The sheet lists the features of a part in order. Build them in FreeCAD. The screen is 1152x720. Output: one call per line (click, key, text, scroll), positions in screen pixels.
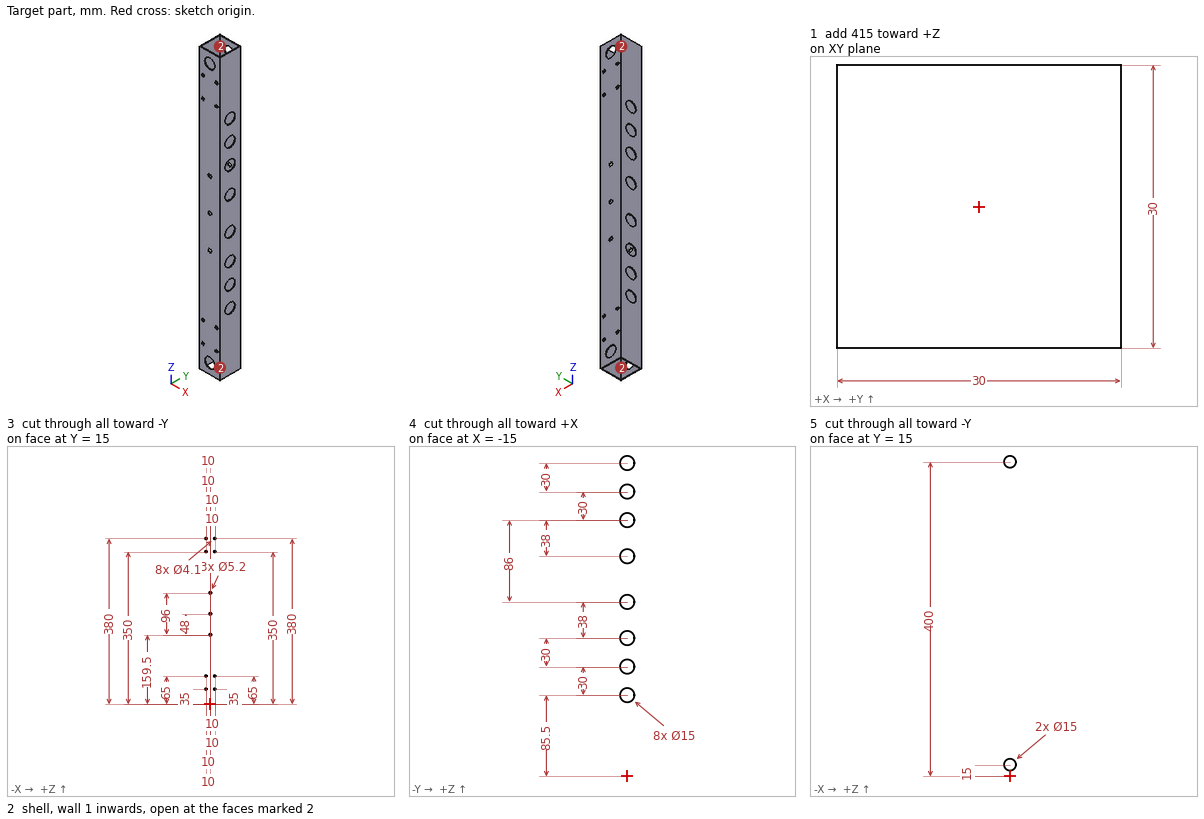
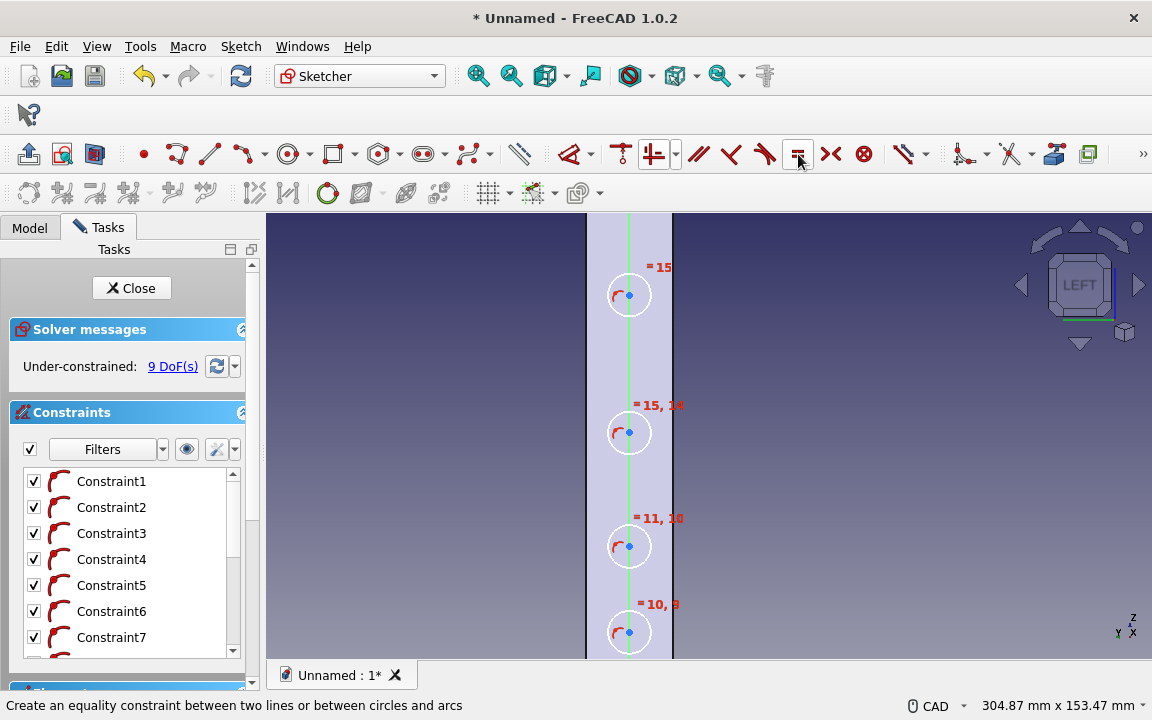
scroll(645, 419, down, 6)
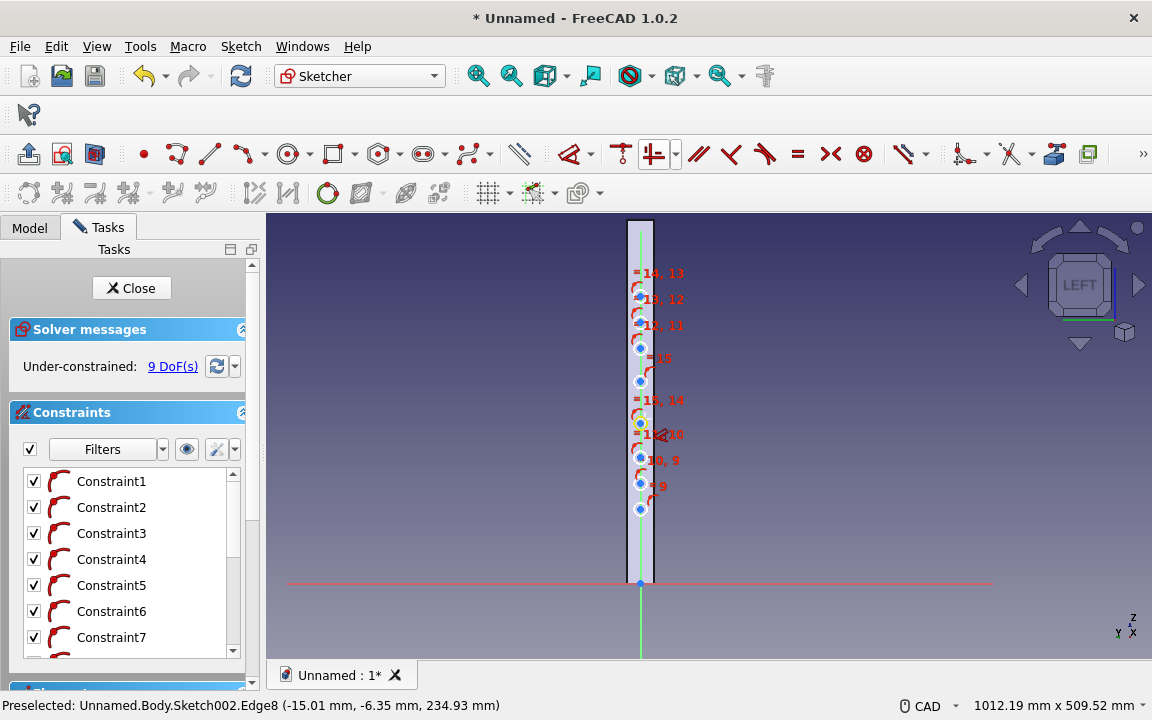
scroll(645, 505, up, 6)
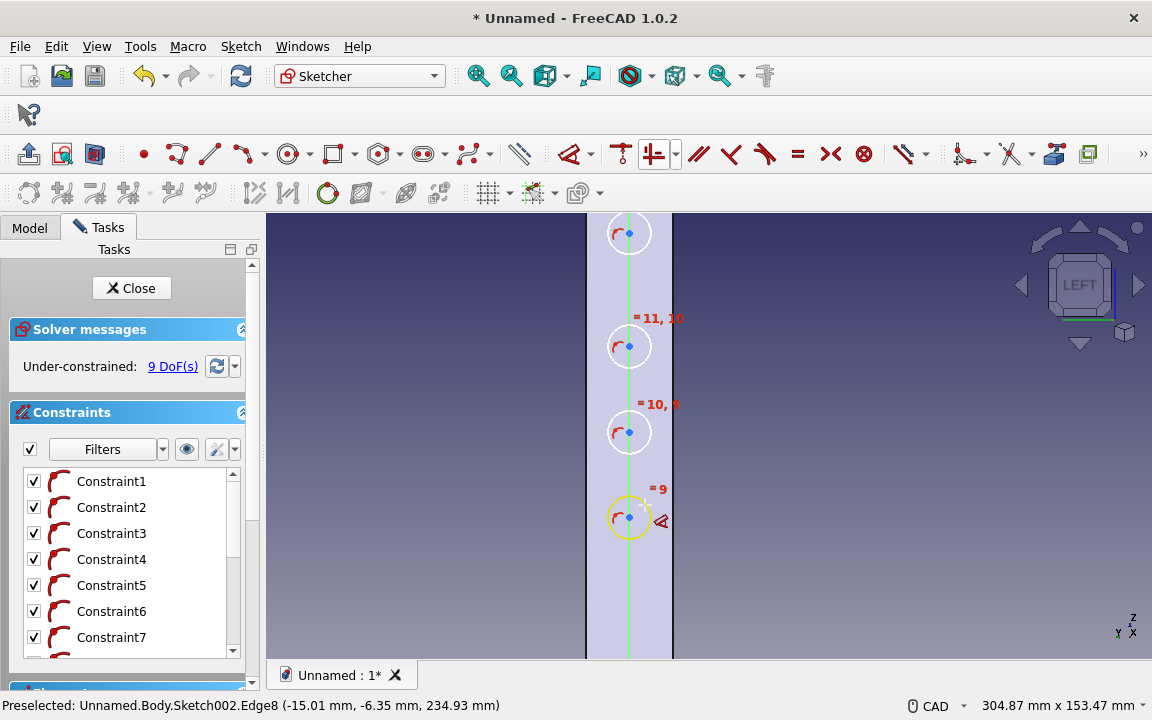
click(645, 503)
click(668, 481)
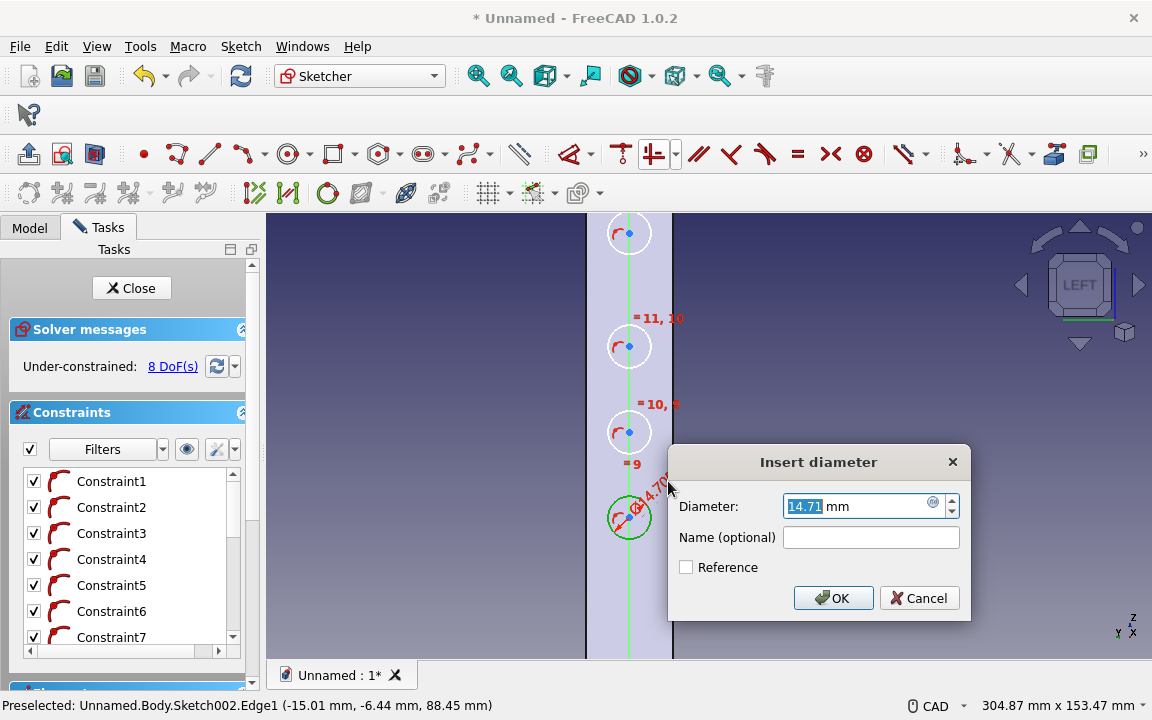
text(15)
key(Return)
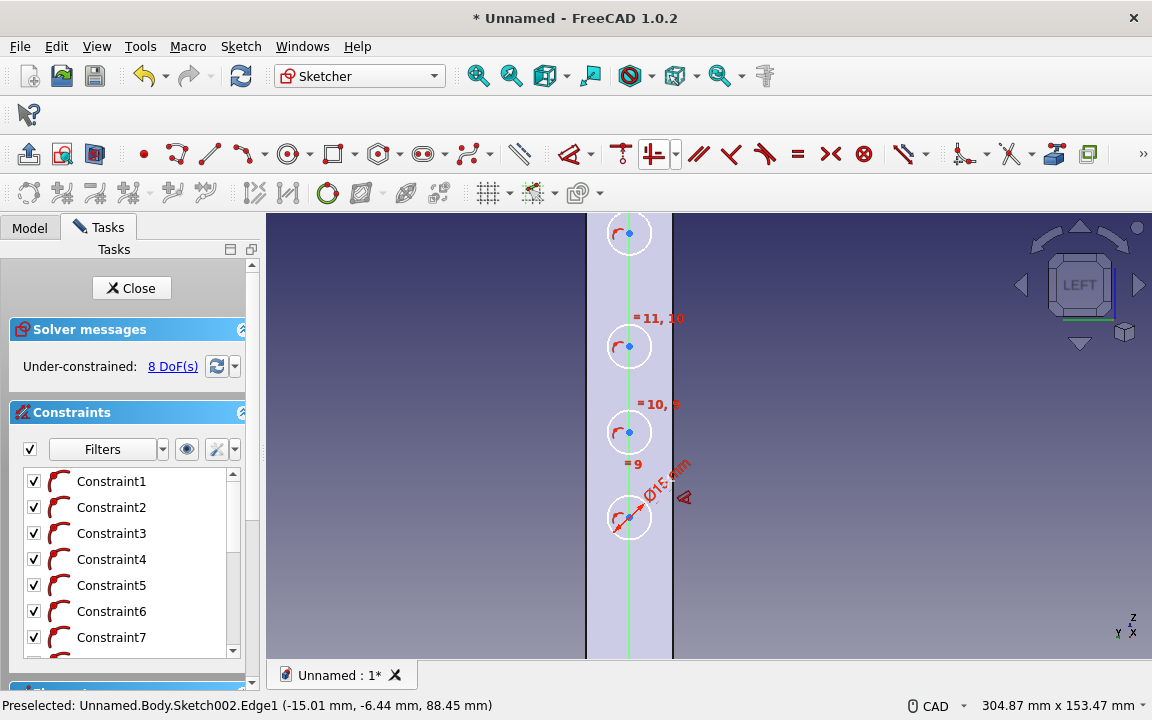
click(629, 518)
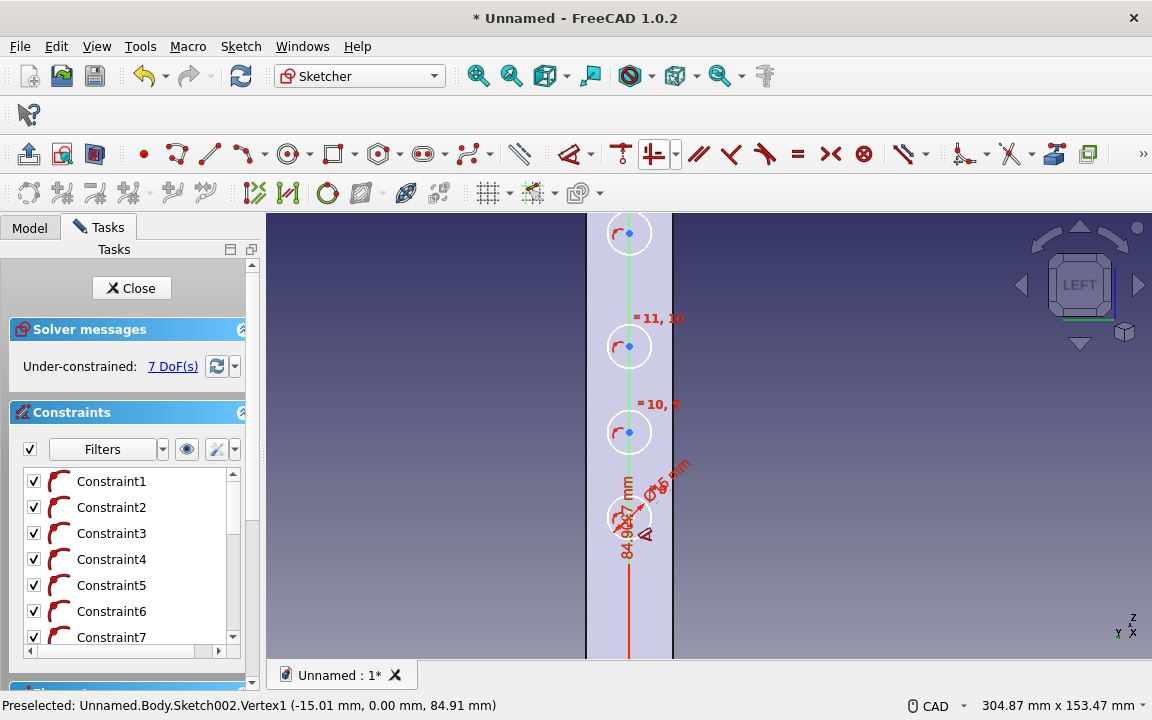
click(629, 432)
click(663, 455)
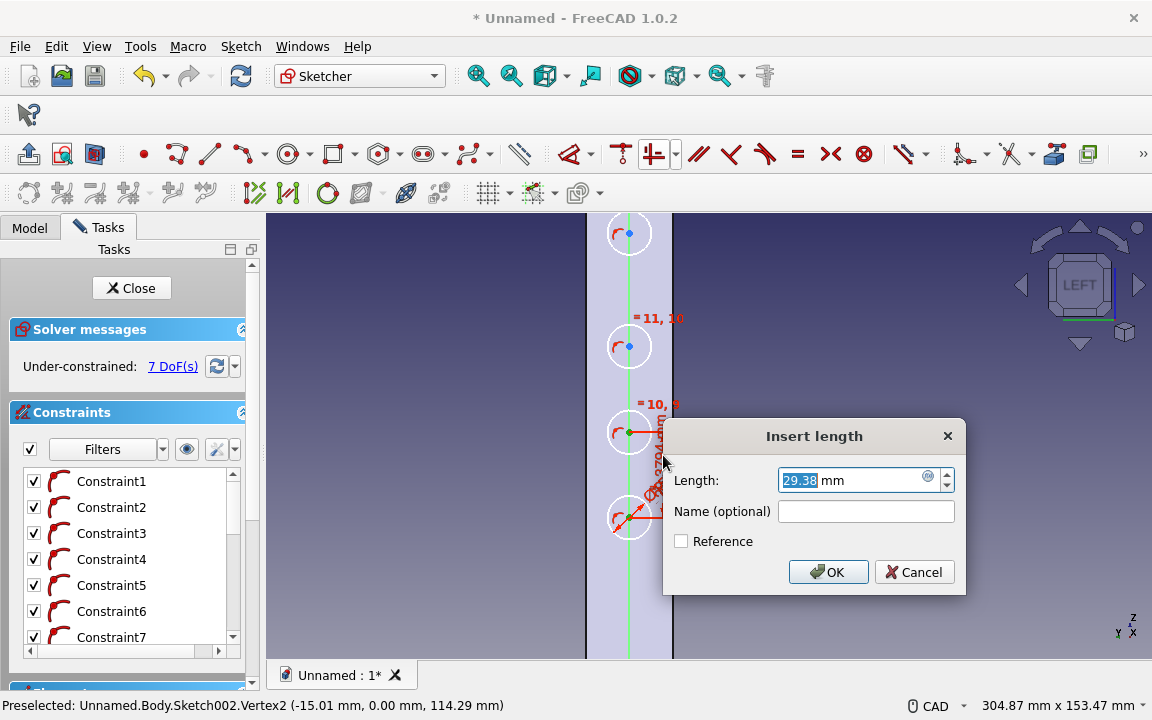
text(30)
key(Return)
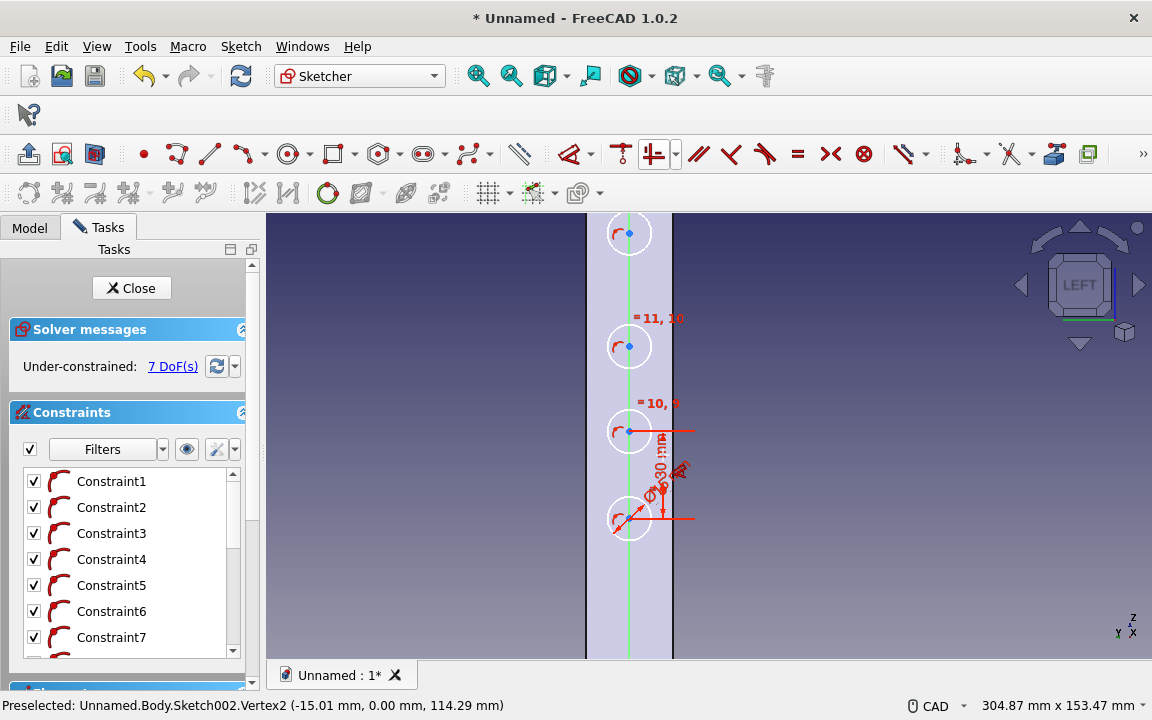
click(629, 431)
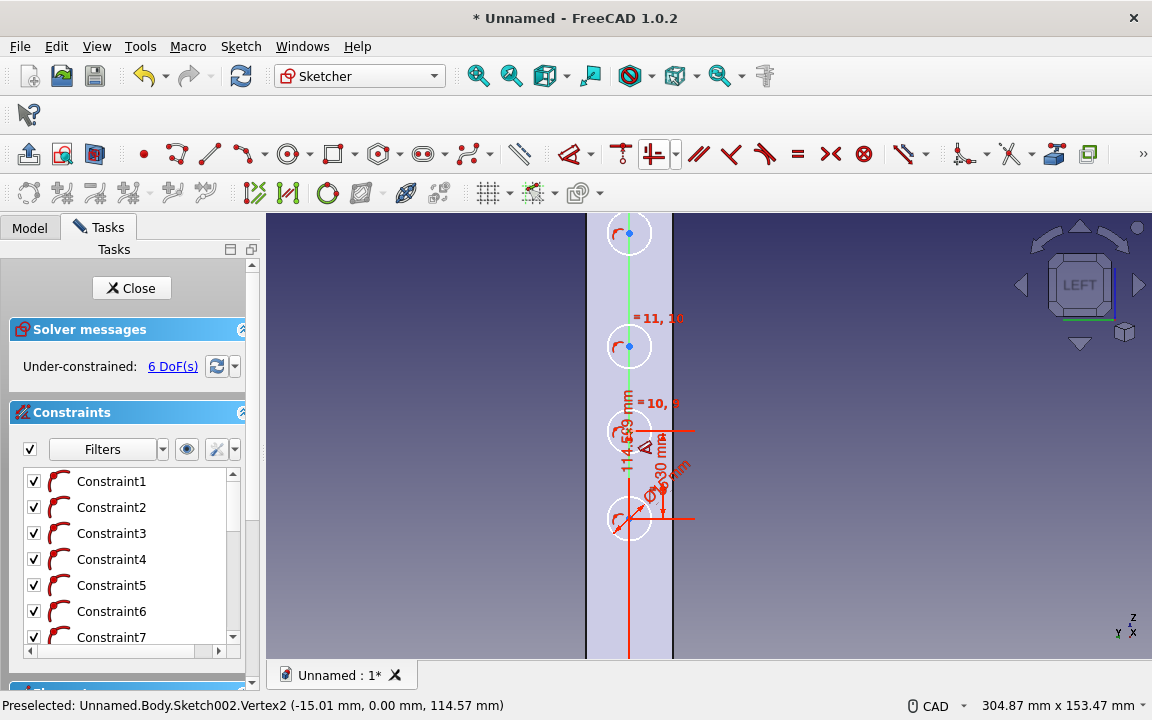
click(629, 347)
click(663, 389)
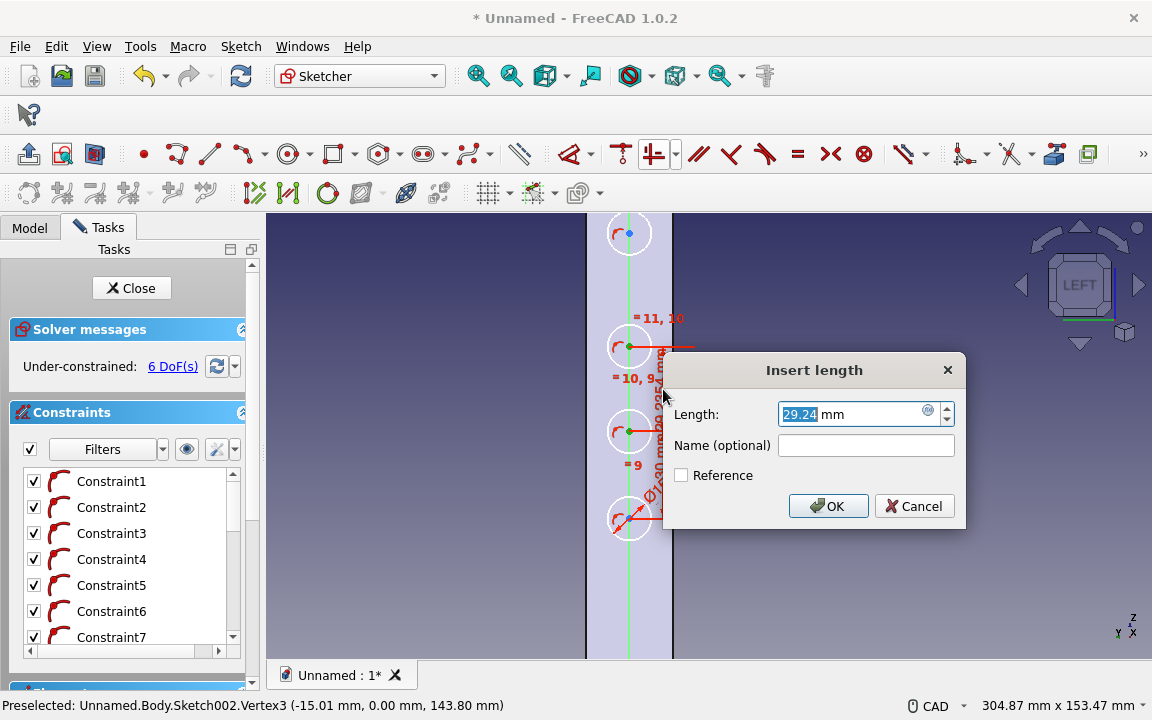
text(30)
key(Return)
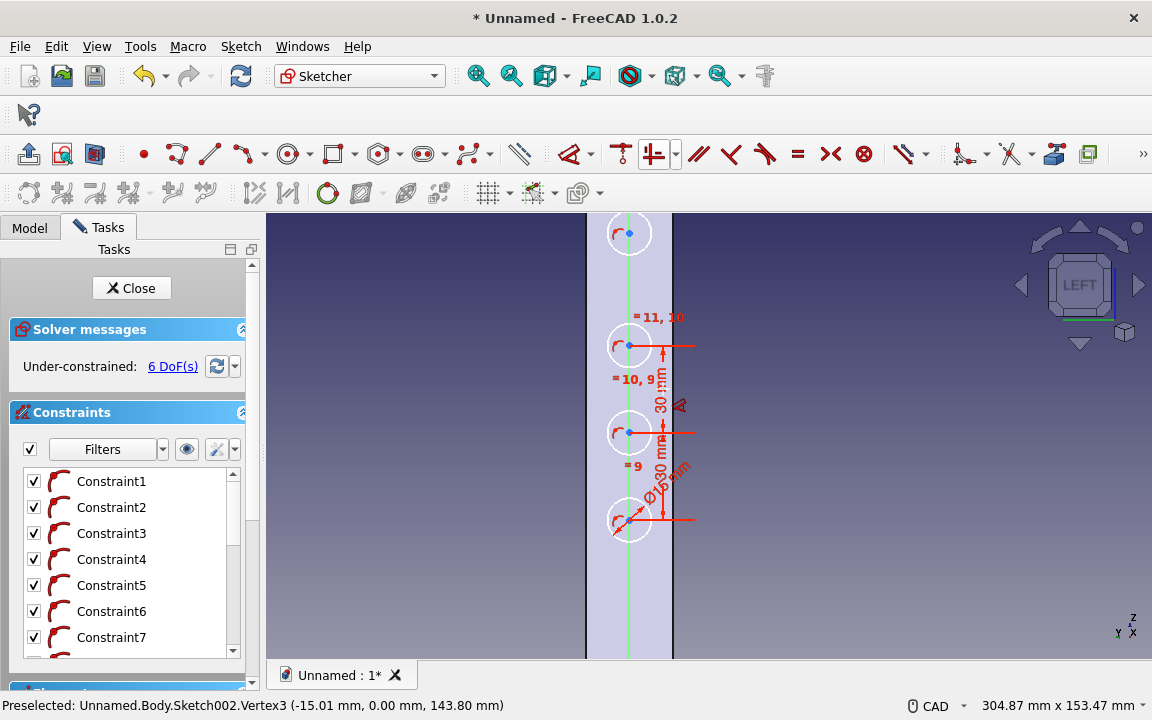
scroll(645, 506, down, 6)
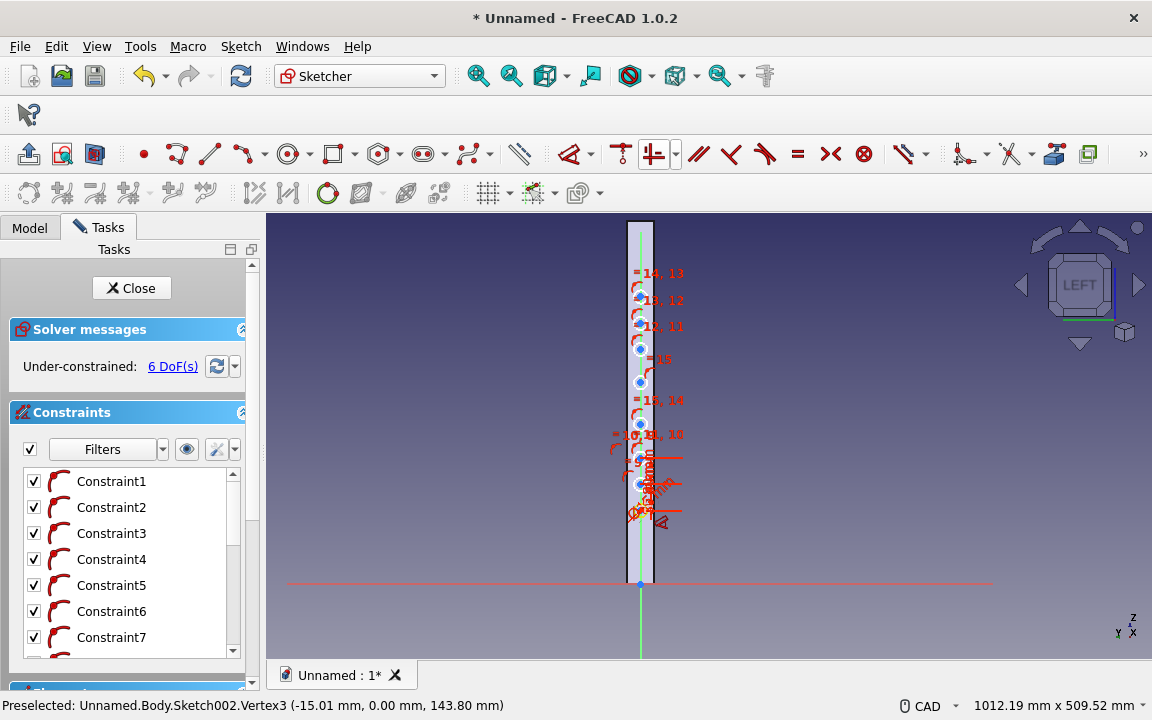
scroll(641, 349, up, 3)